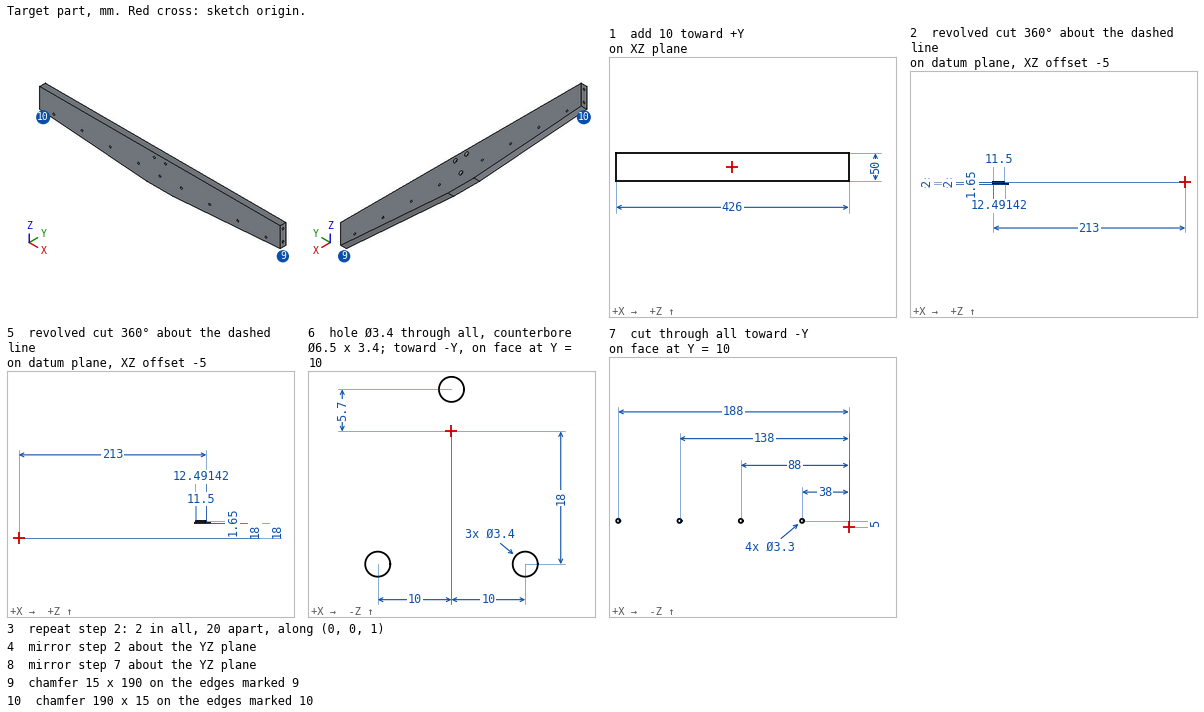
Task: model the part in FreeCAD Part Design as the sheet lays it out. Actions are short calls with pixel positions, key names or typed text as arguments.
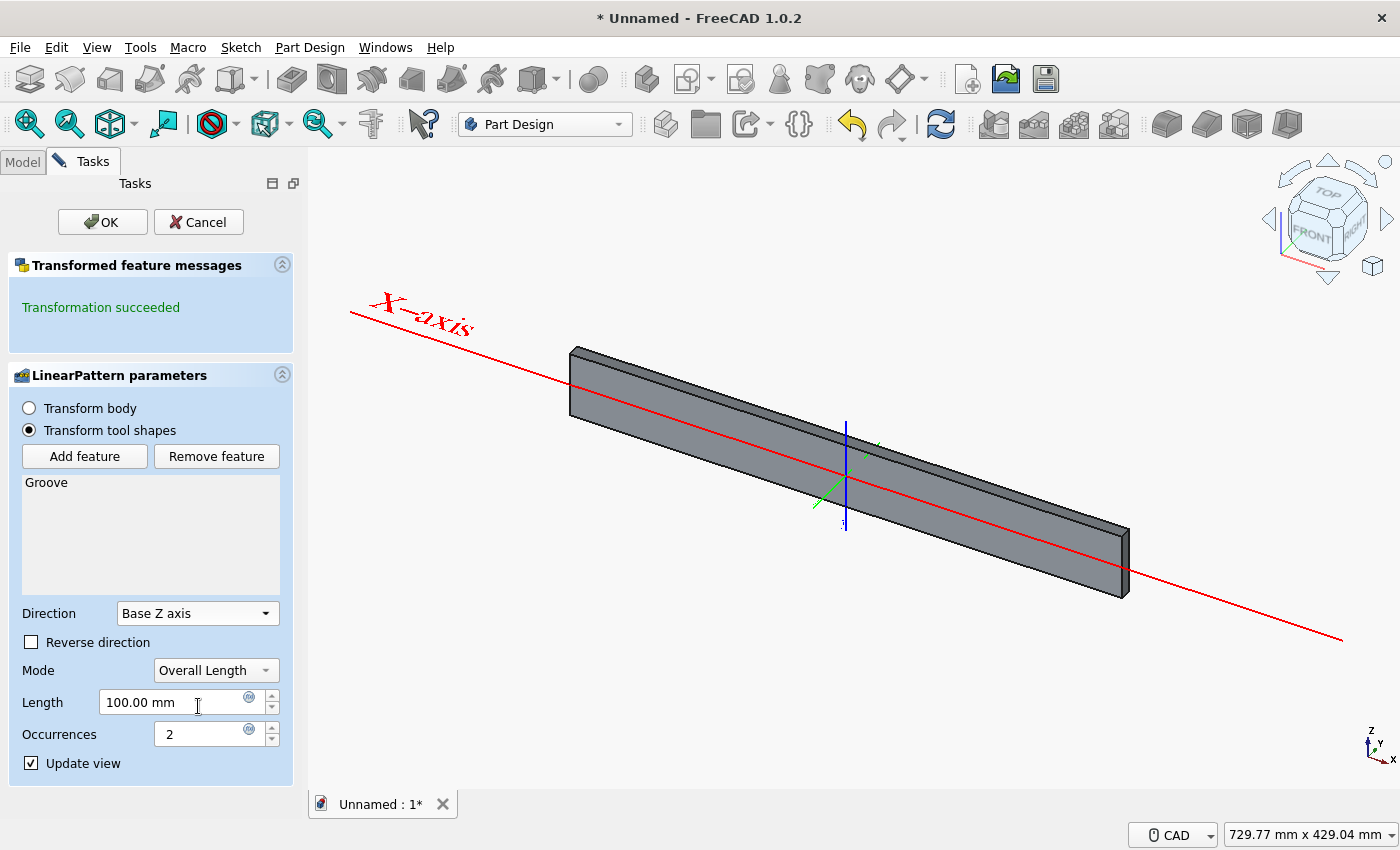
click(217, 670)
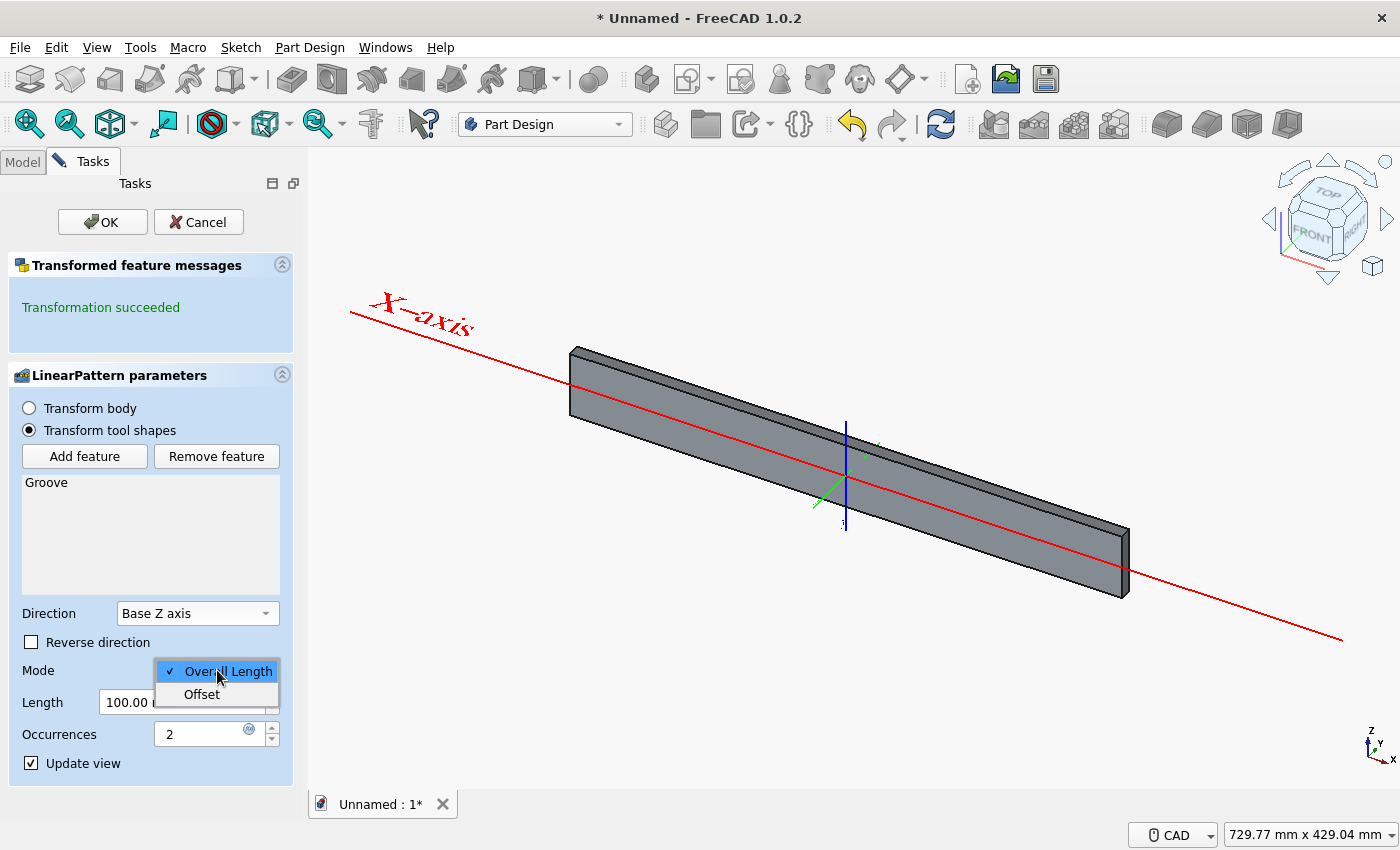
click(216, 694)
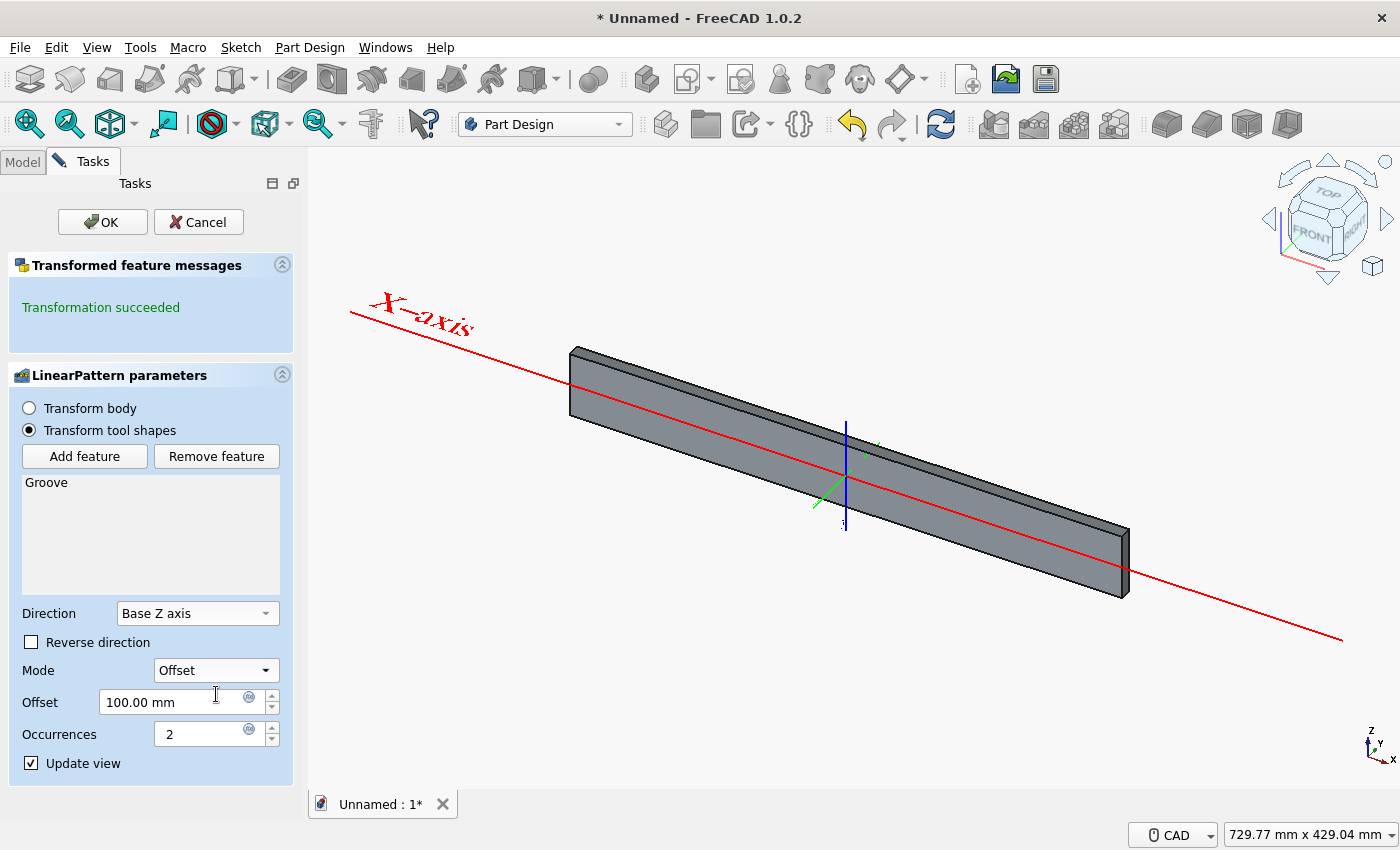
triple_click(182, 702)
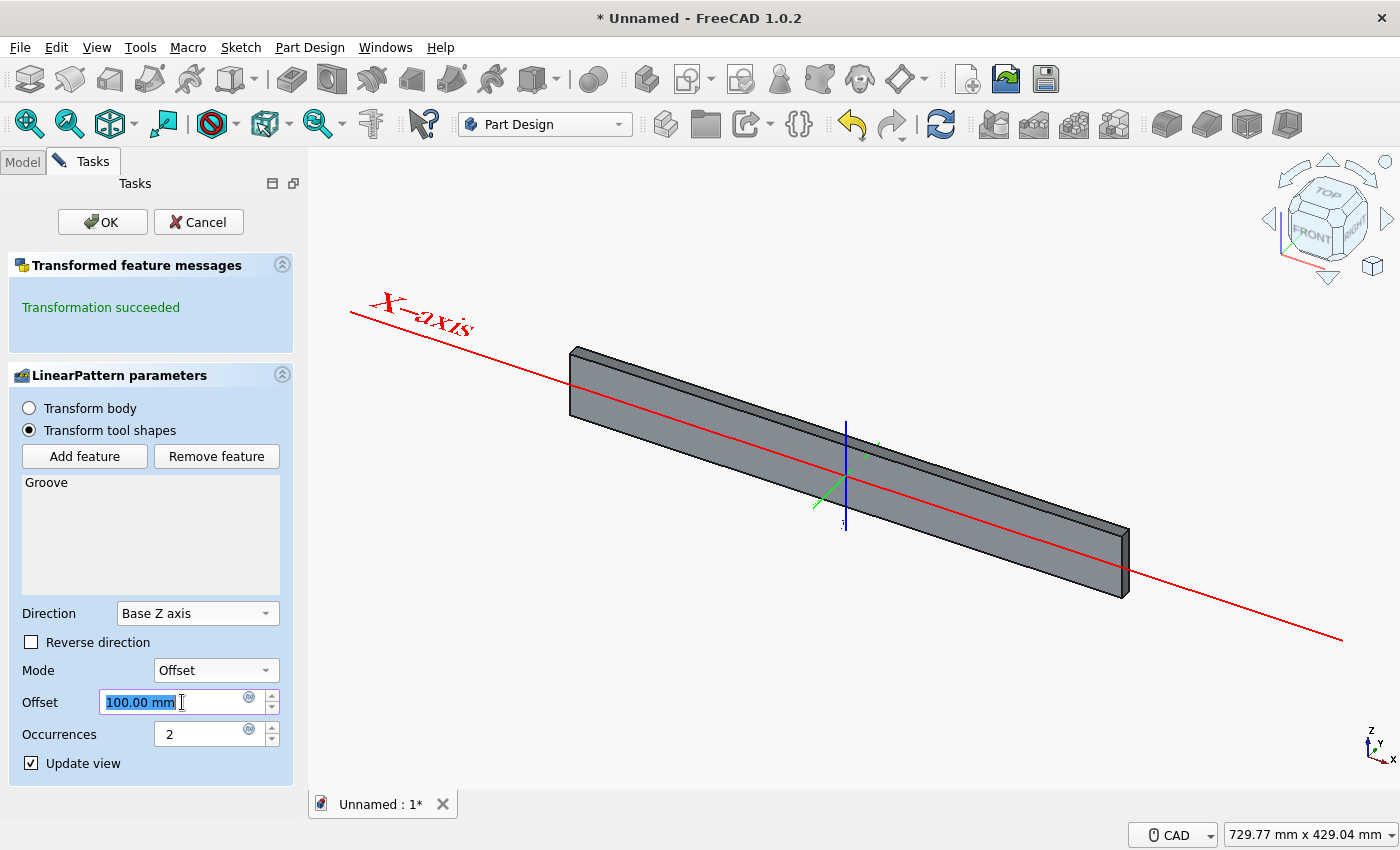
text(20)
key(Tab)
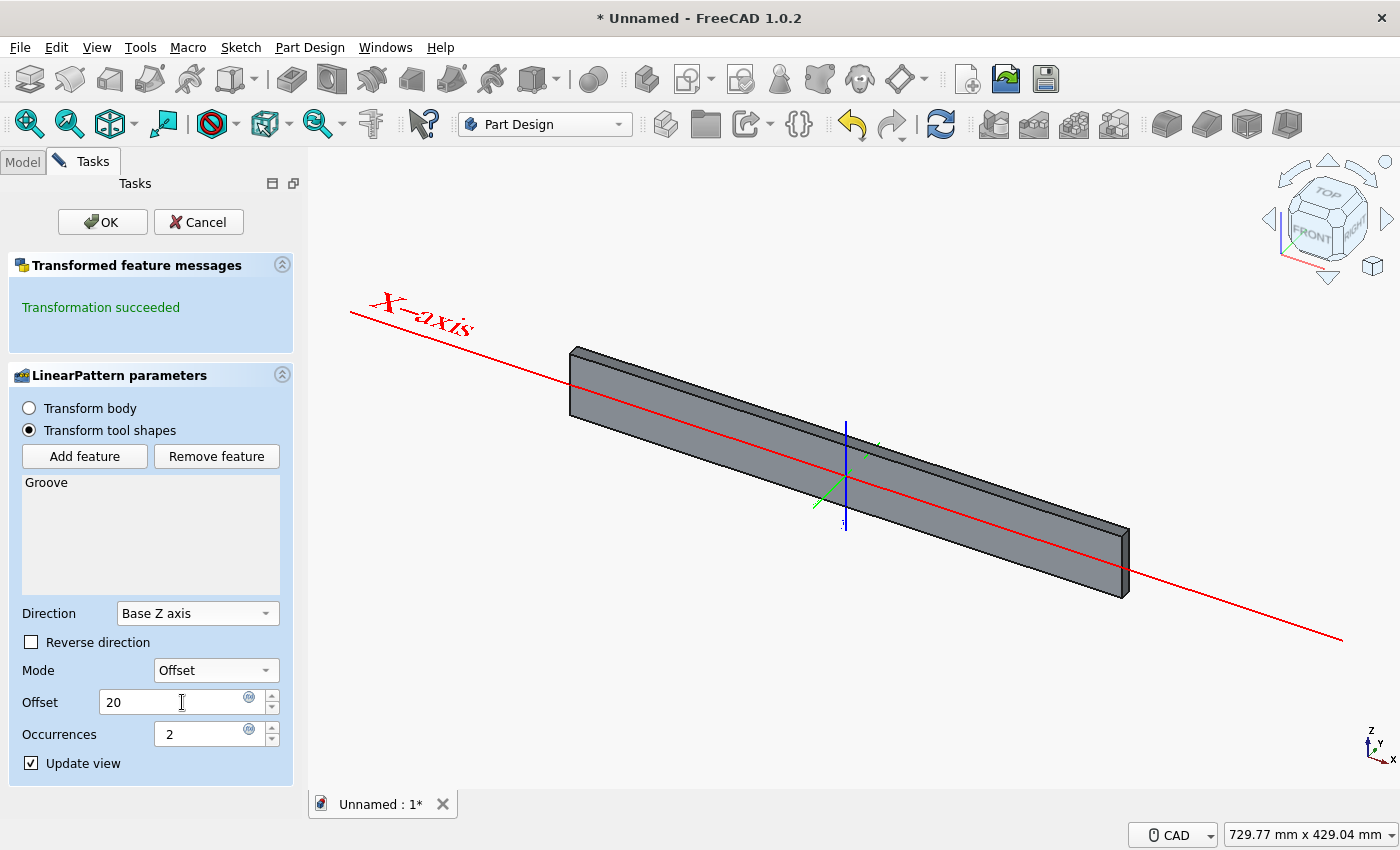
triple_click(209, 734)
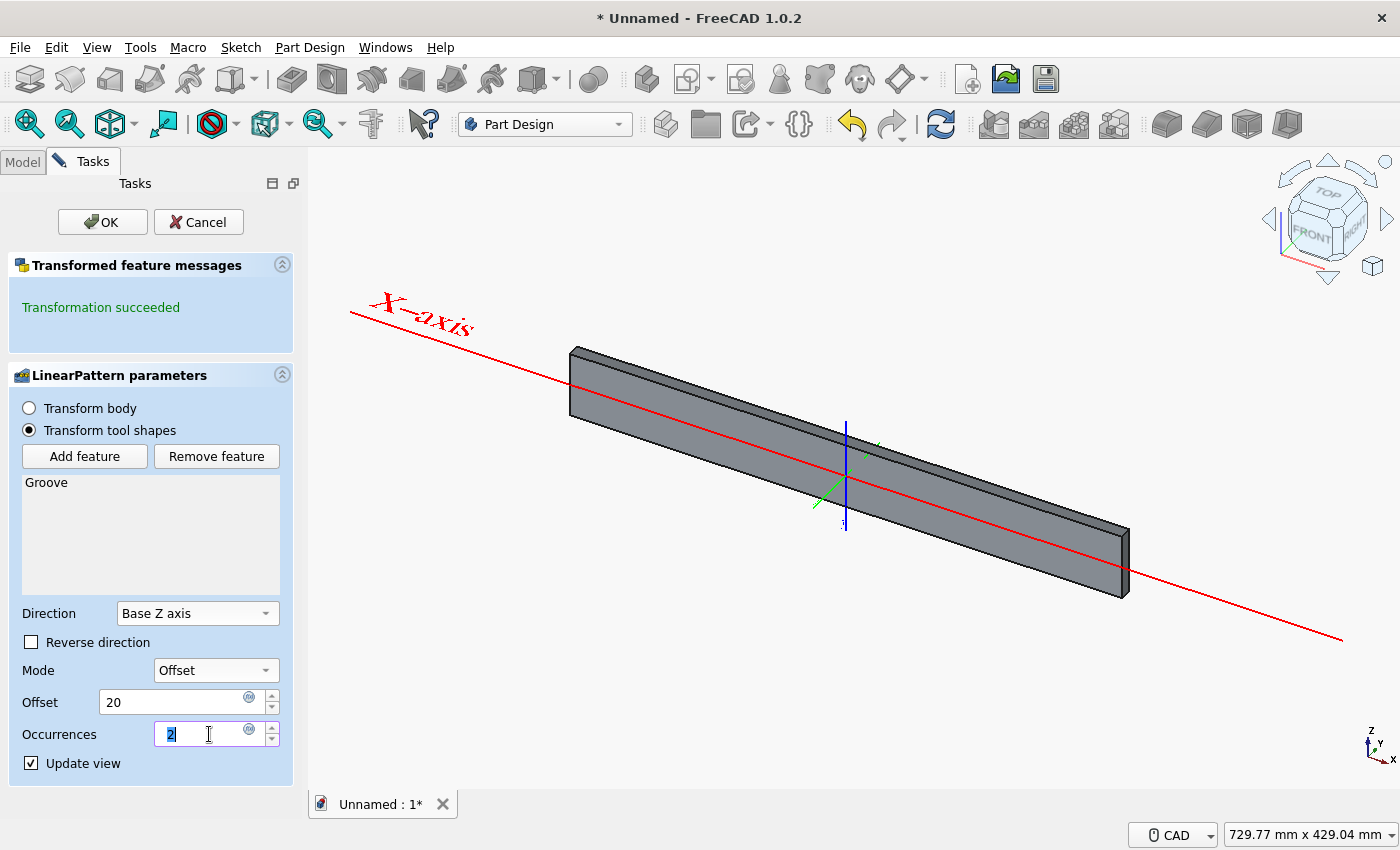
text(2)
key(Tab)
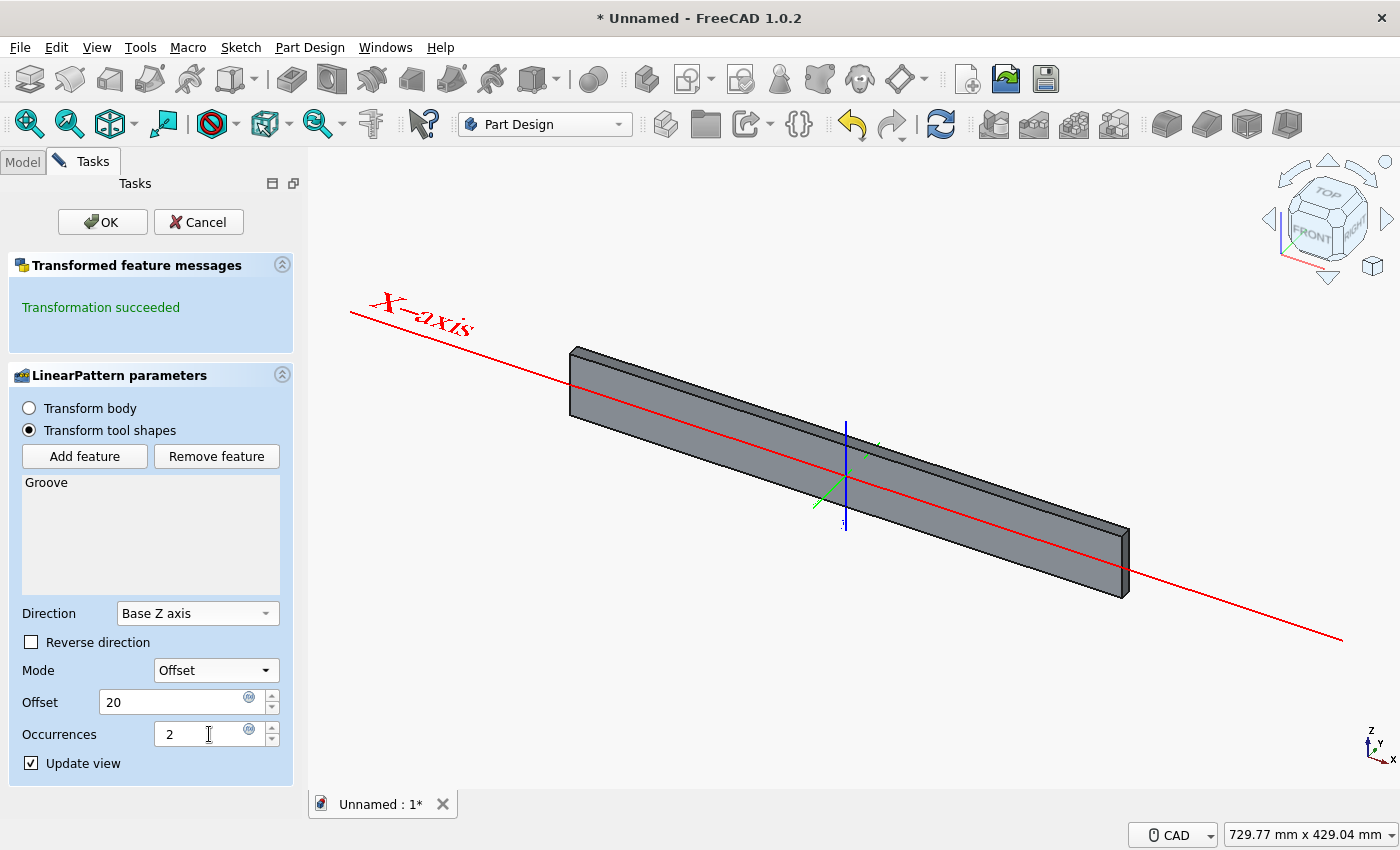
click(103, 222)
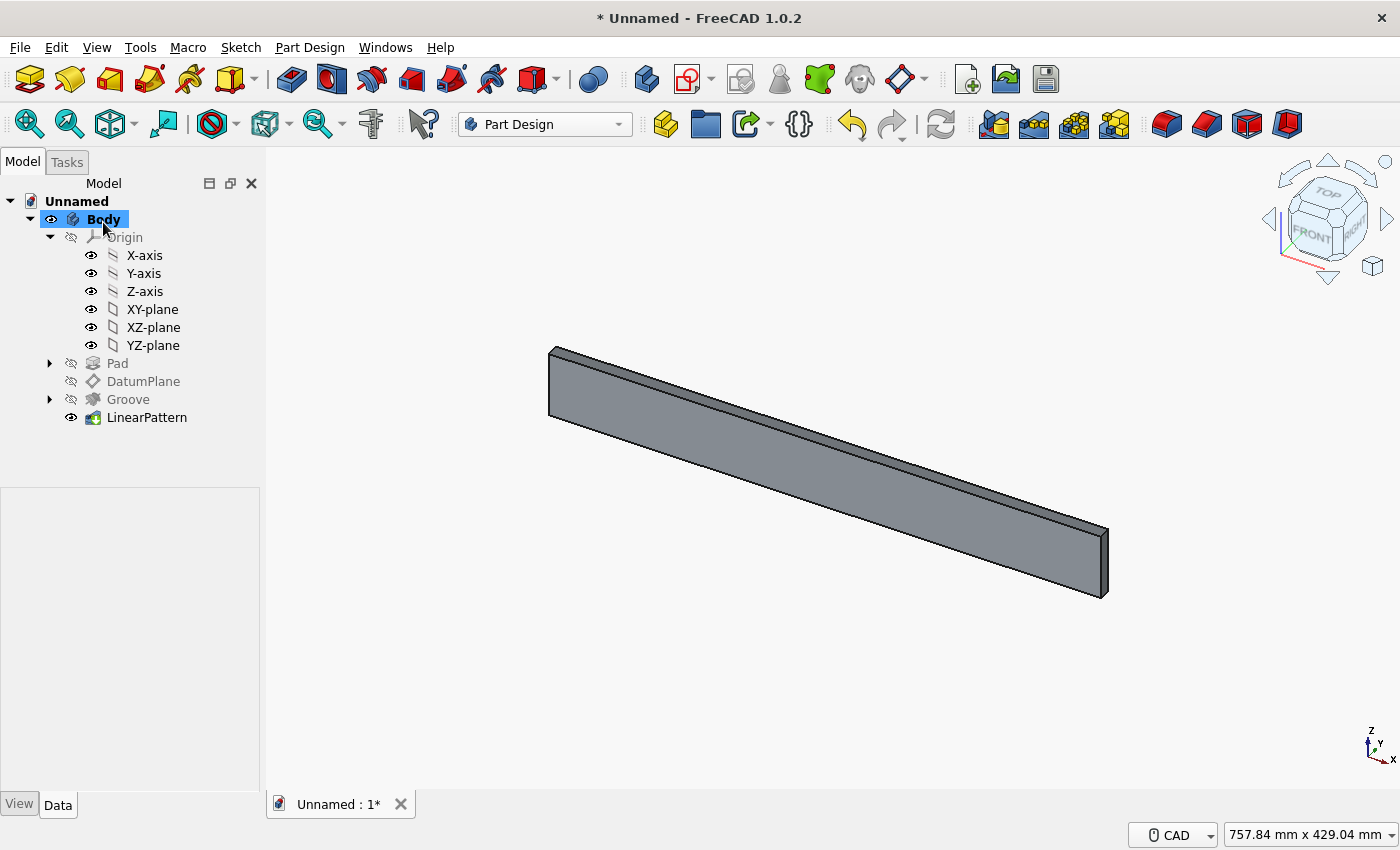
click(116, 399)